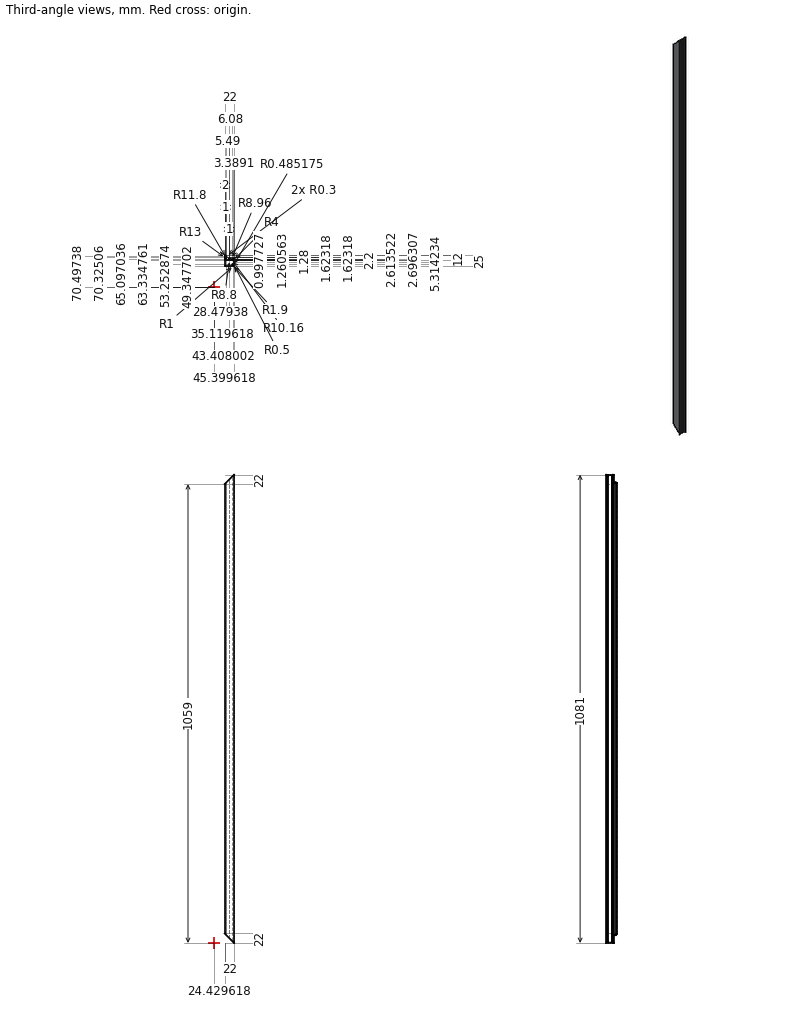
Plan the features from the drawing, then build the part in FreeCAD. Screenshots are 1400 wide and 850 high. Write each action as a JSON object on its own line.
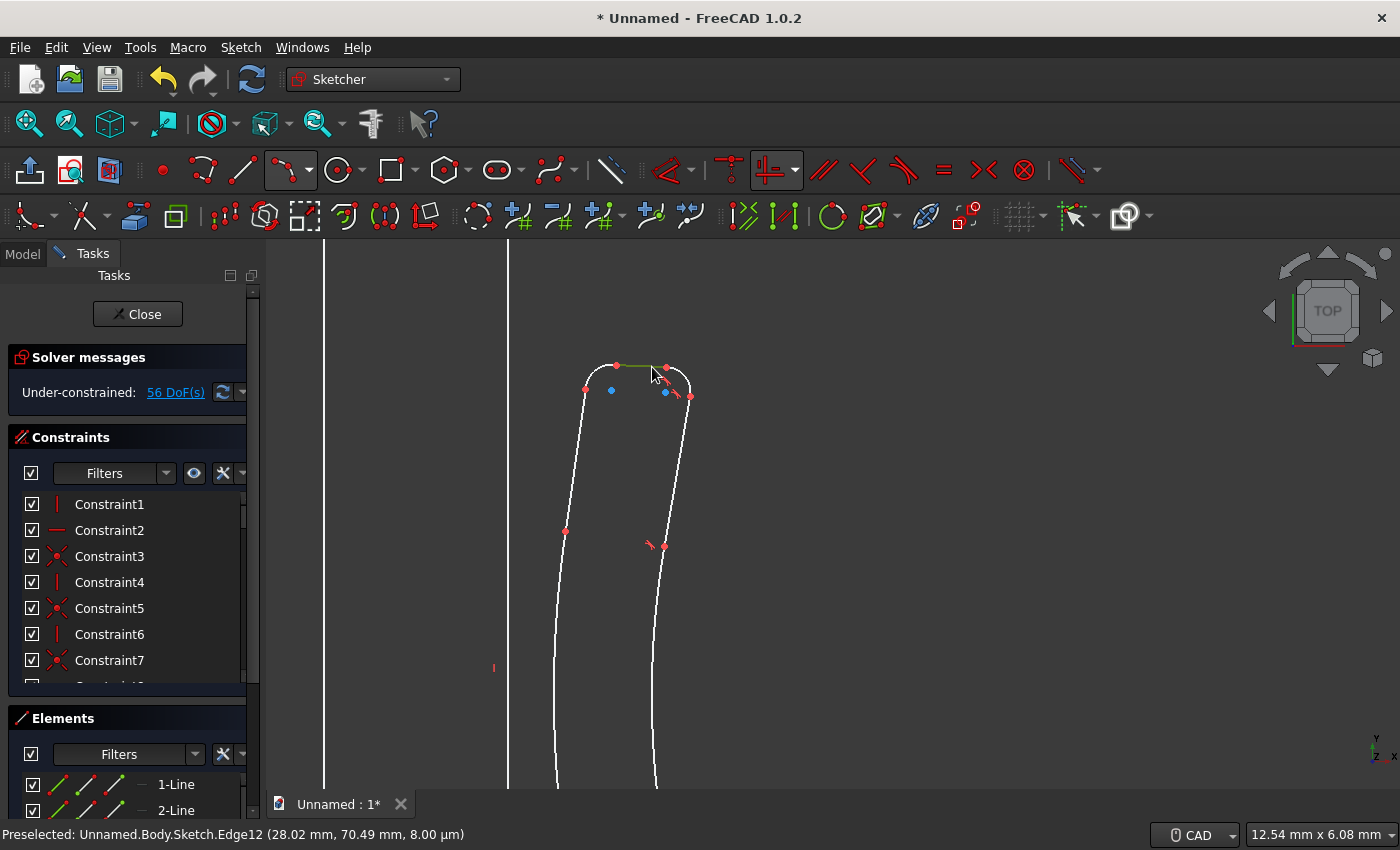
{"action": "left_click", "coordinate": [604, 366]}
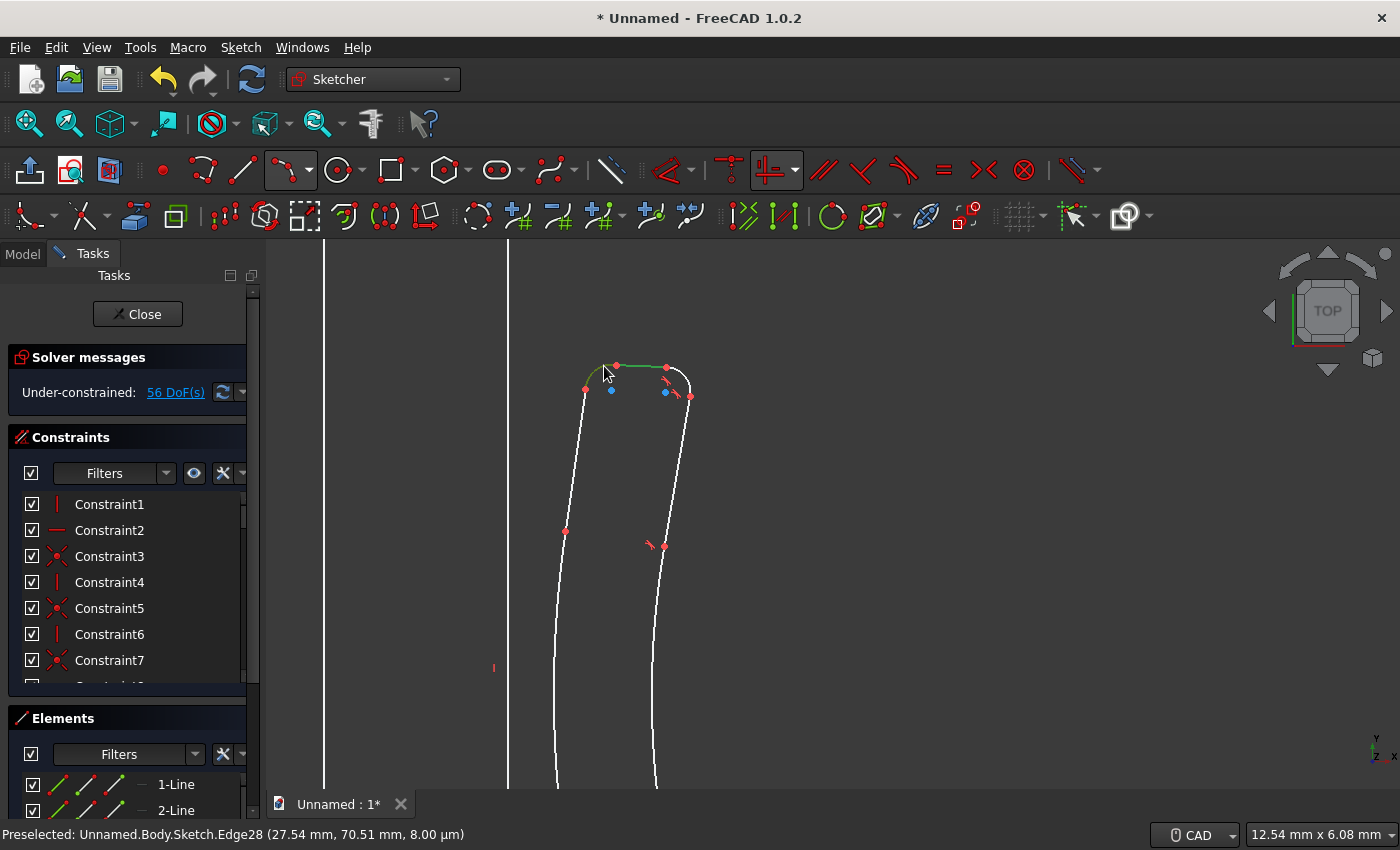
{"action": "left_click", "coordinate": [904, 170]}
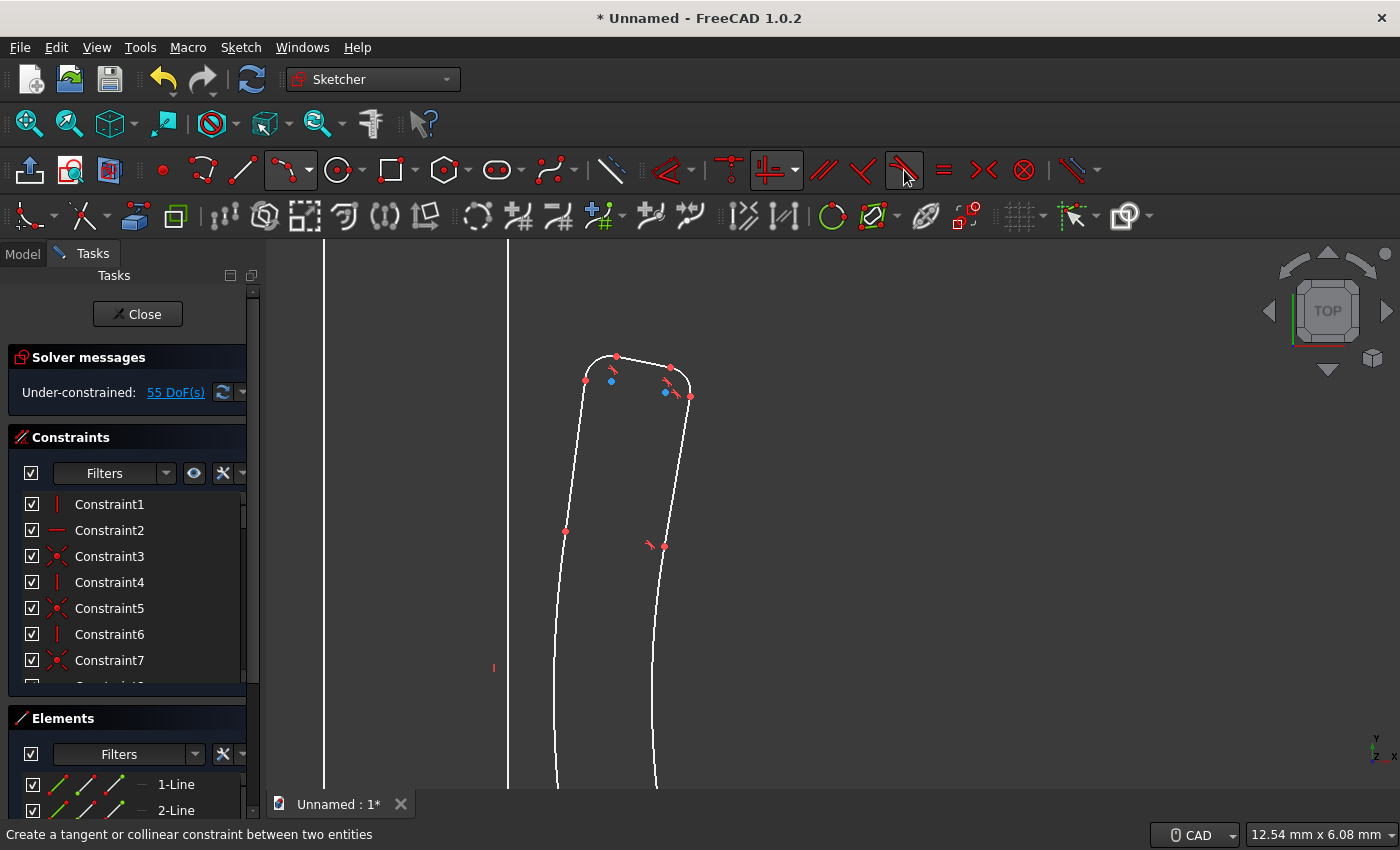
{"action": "scroll", "coordinate": [654, 368], "scroll_direction": "down", "scroll_amount": 9}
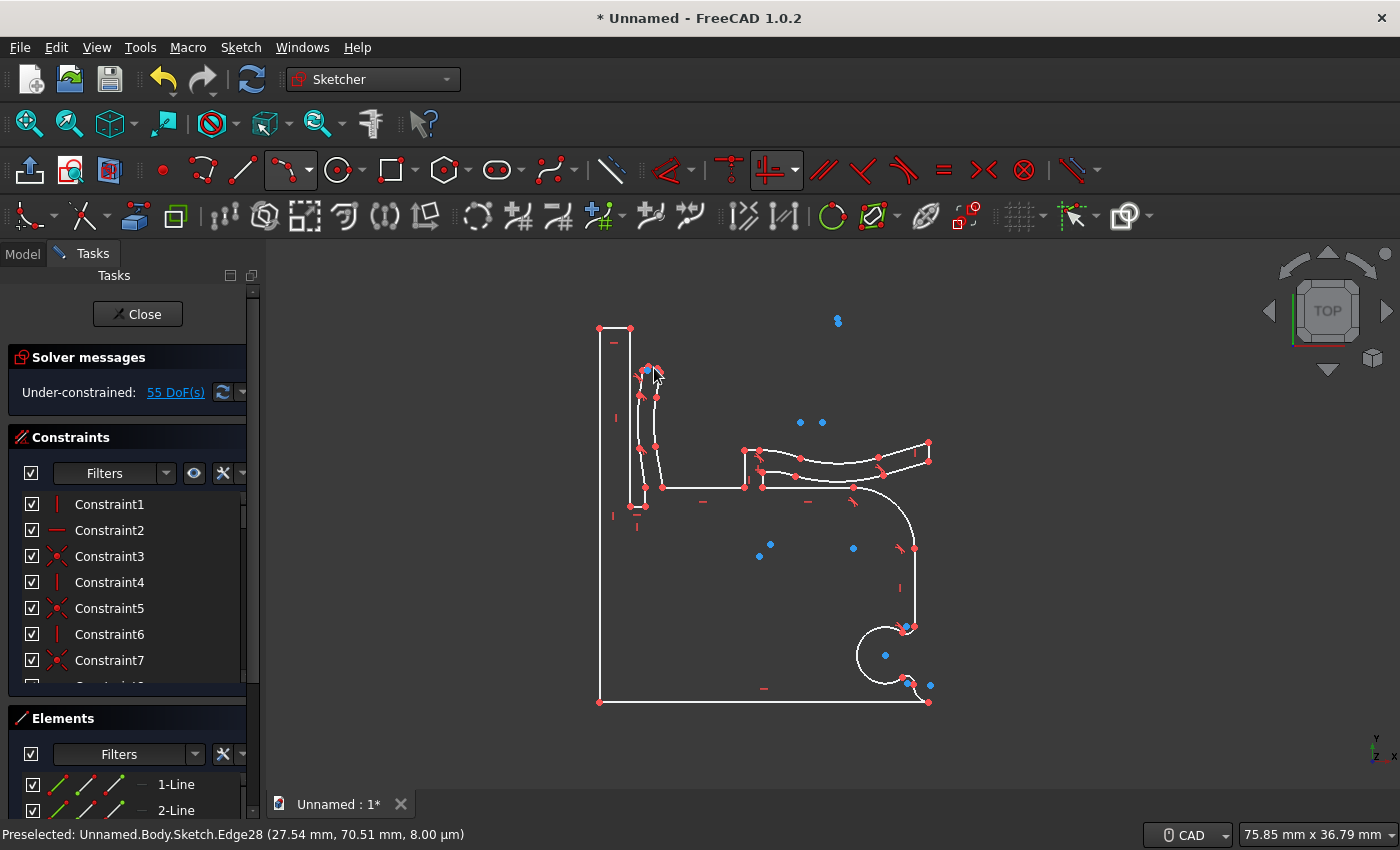
{"action": "scroll", "coordinate": [642, 378], "scroll_direction": "up", "scroll_amount": 4}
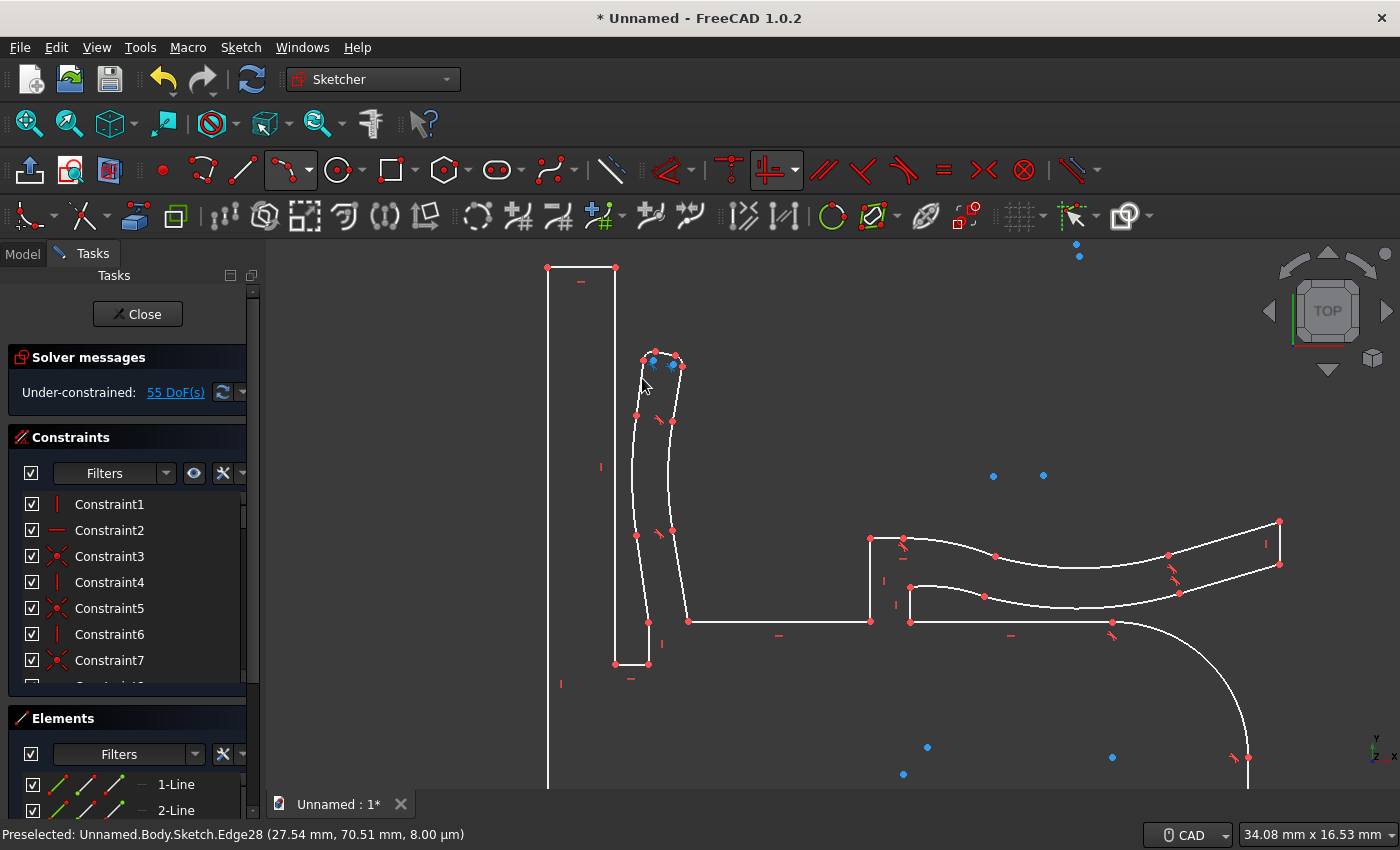
{"action": "left_click", "coordinate": [641, 377]}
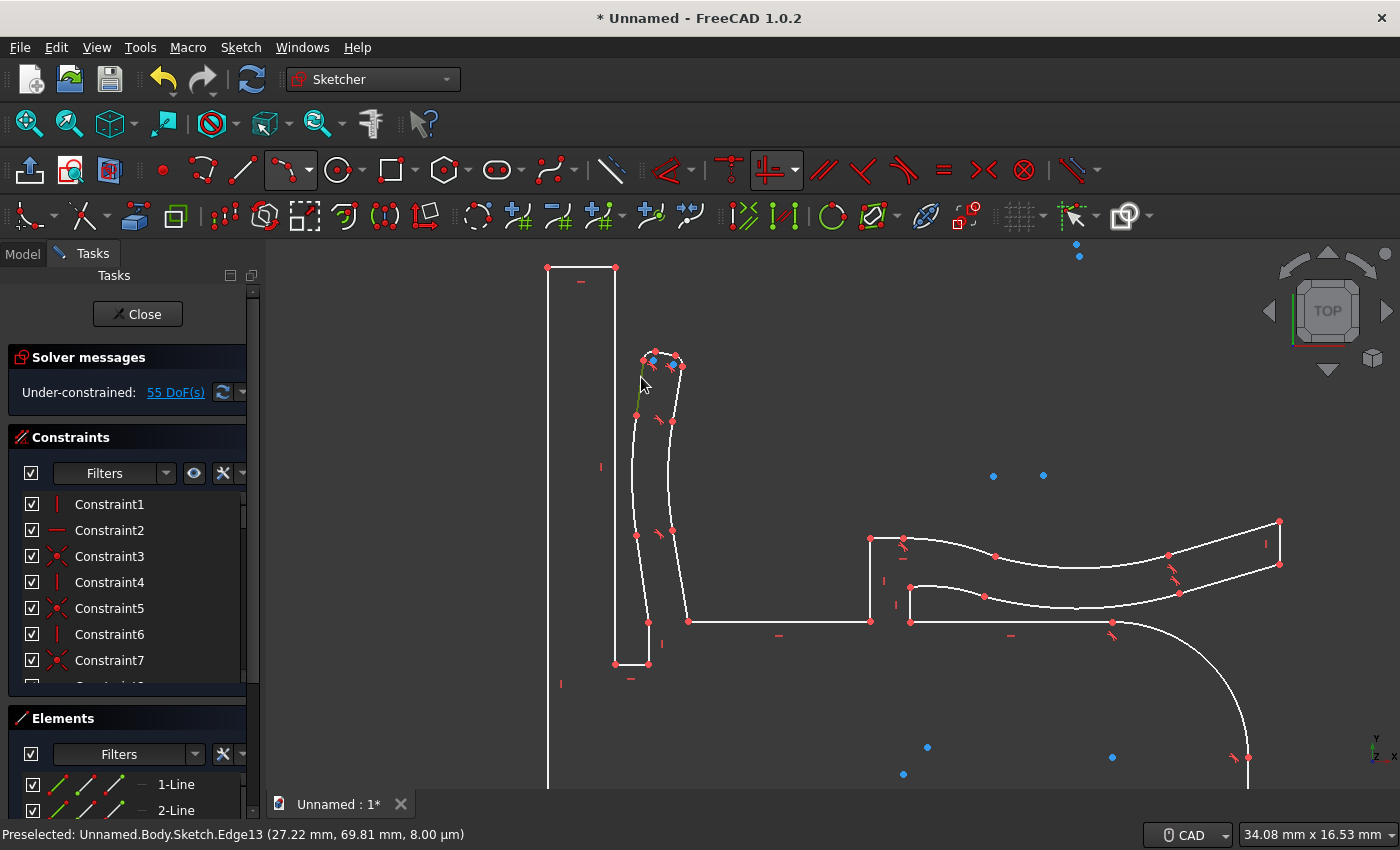
{"action": "scroll", "coordinate": [647, 353], "scroll_direction": "up", "scroll_amount": 3}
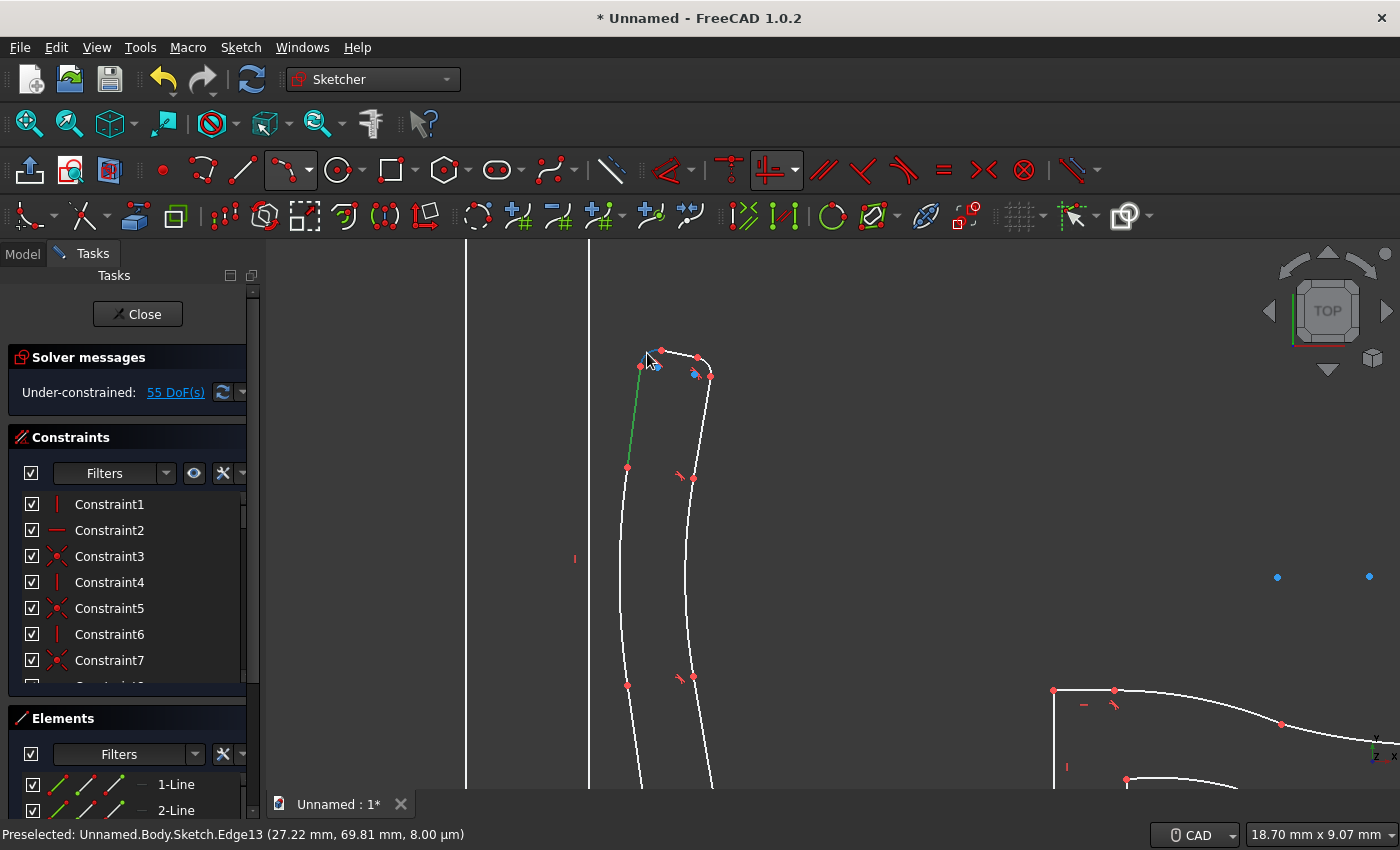
{"action": "left_click", "coordinate": [647, 354]}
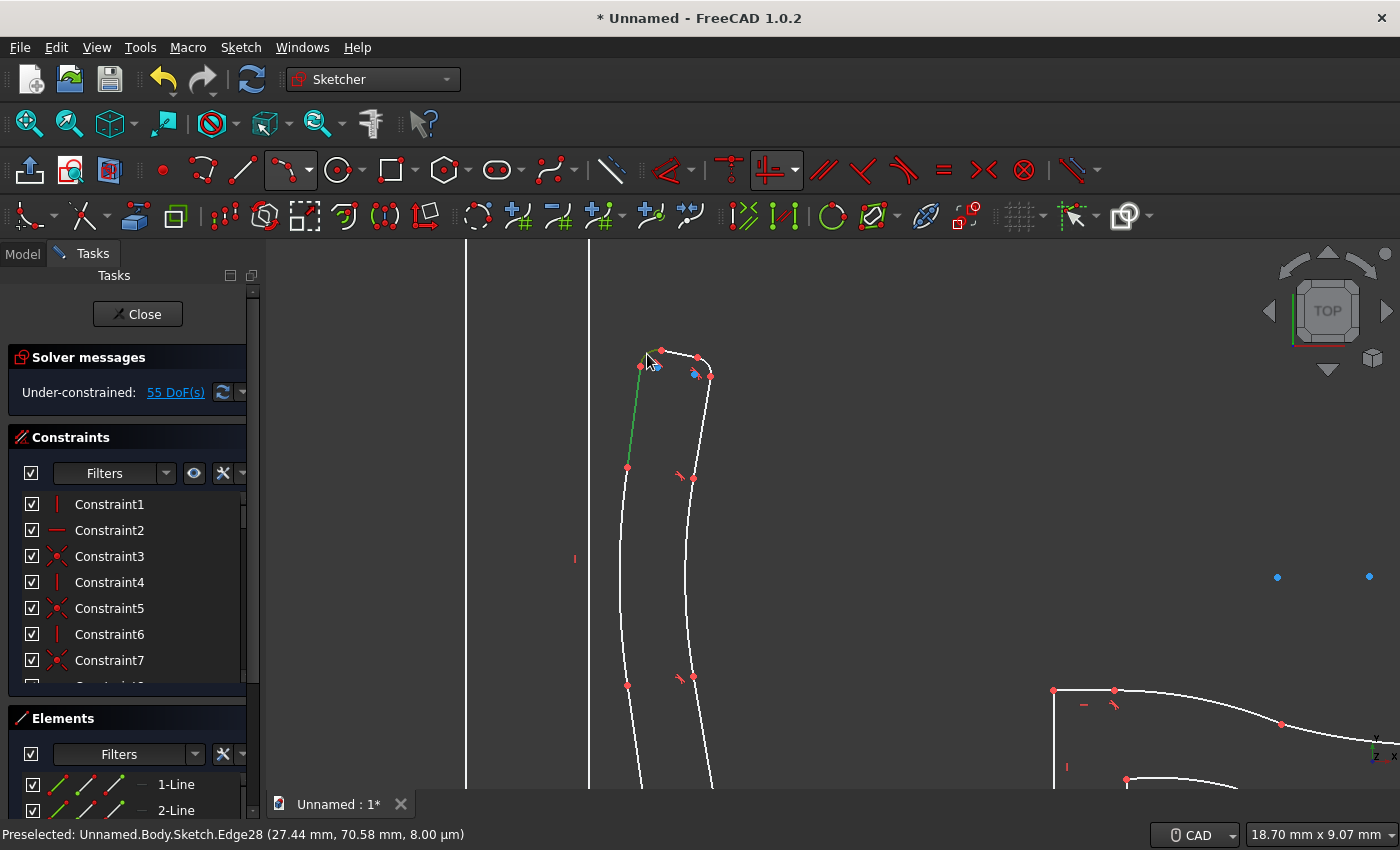
{"action": "left_click", "coordinate": [904, 170]}